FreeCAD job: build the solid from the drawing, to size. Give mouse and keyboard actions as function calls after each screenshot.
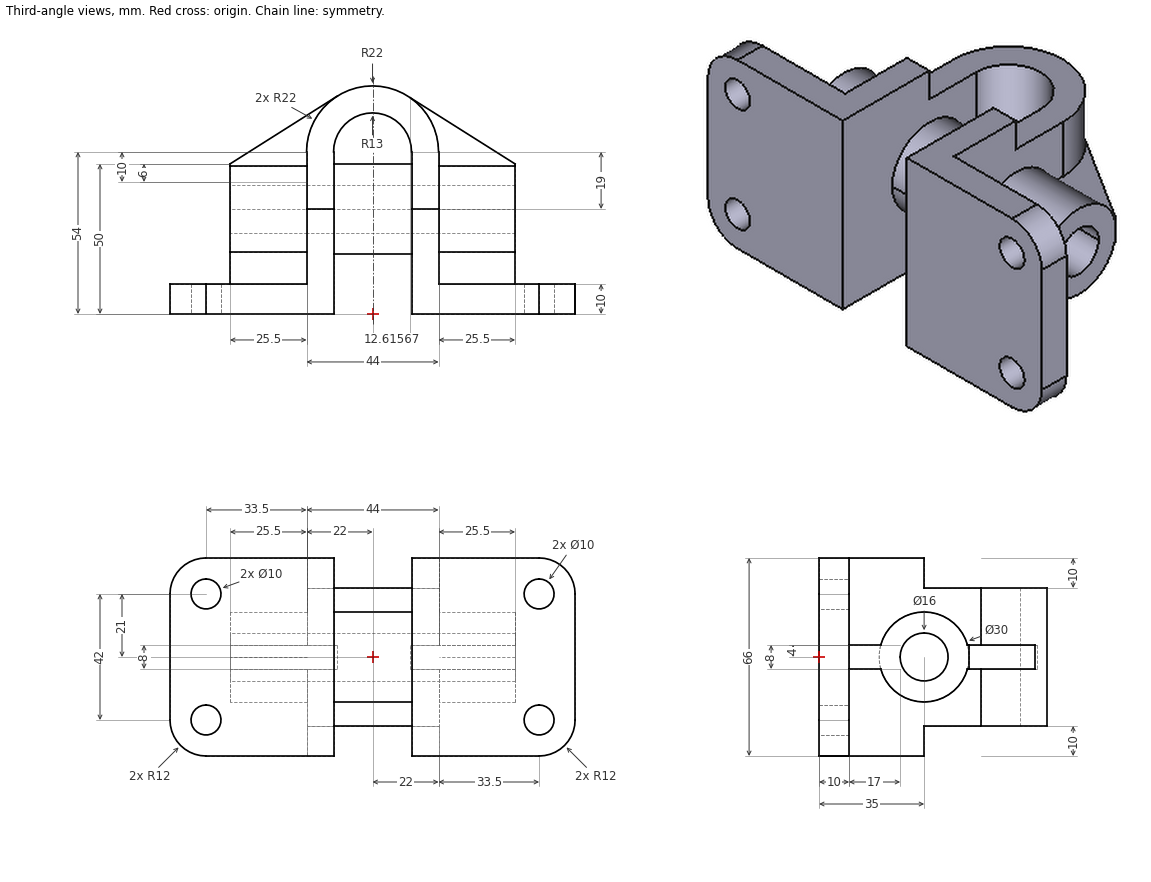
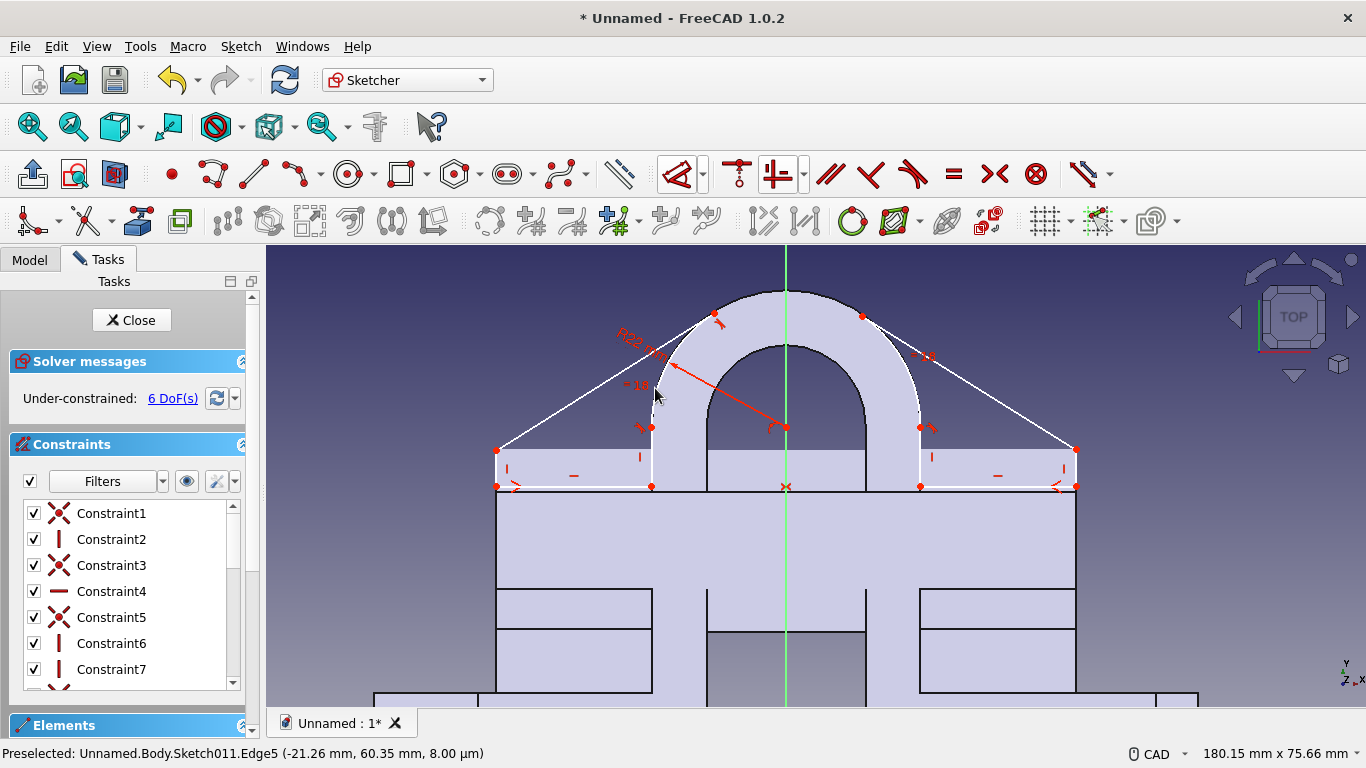
scroll(496, 462, up, 2)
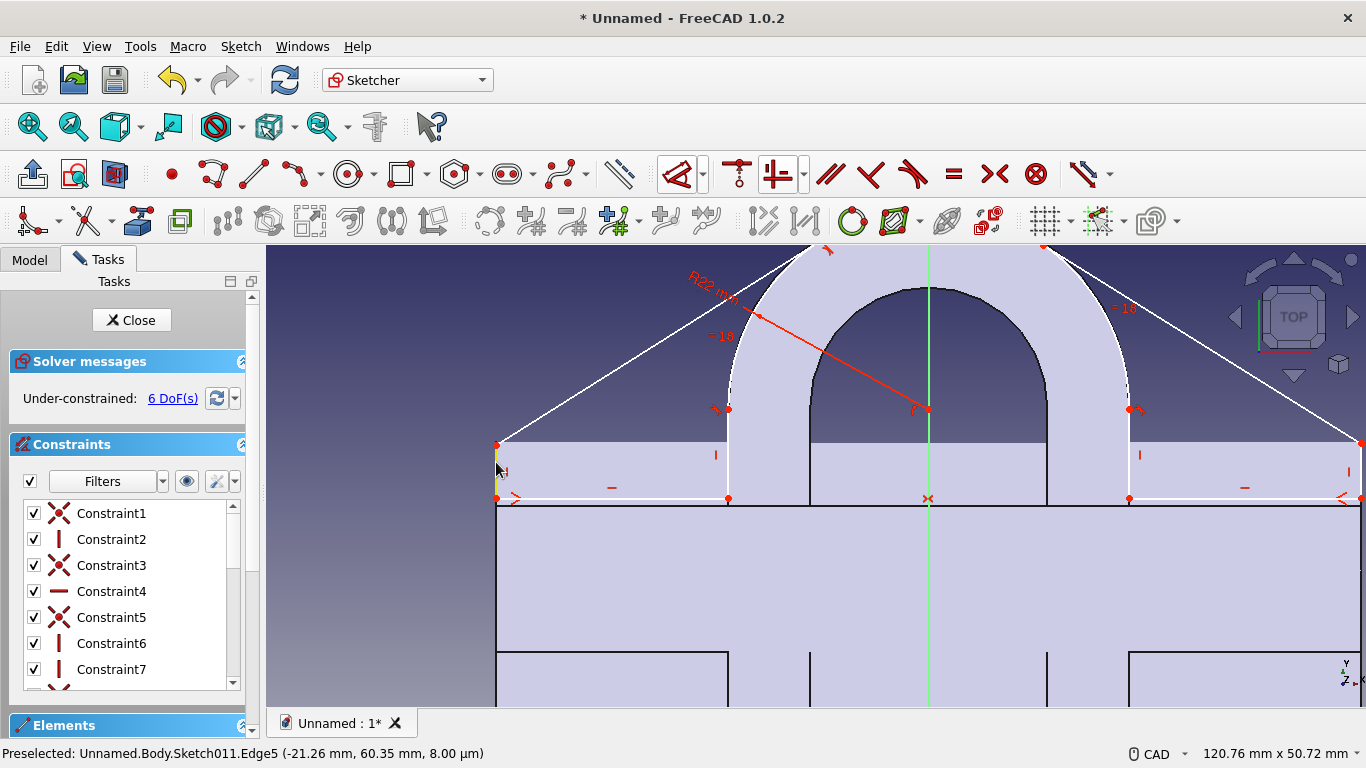
click(496, 461)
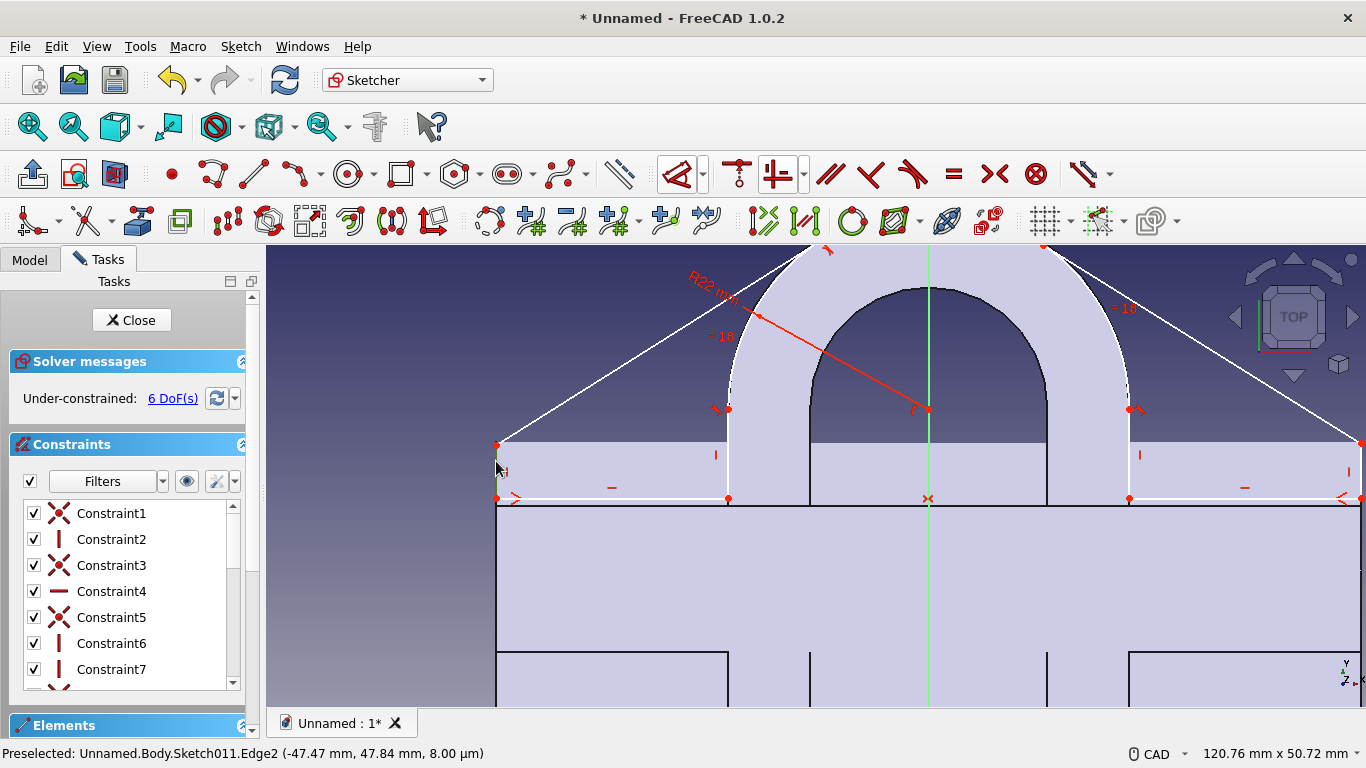
click(702, 174)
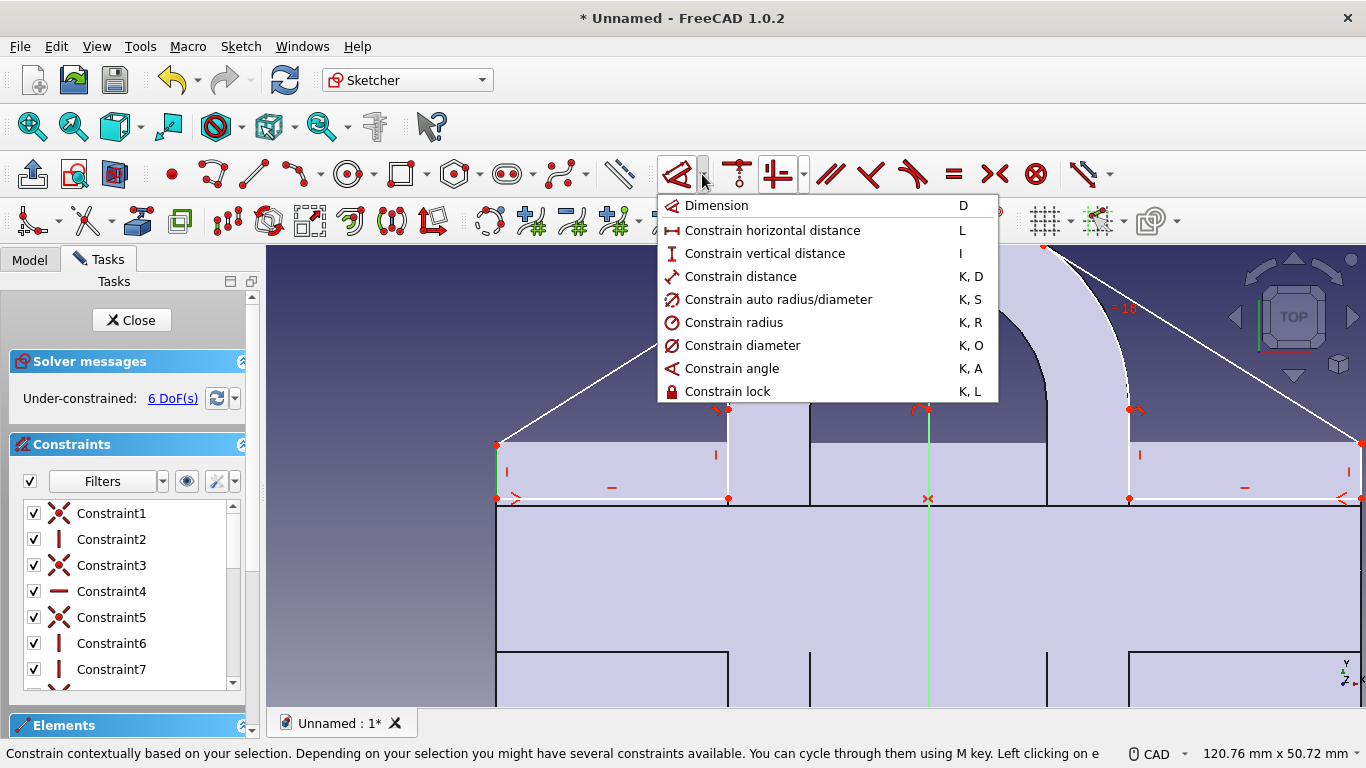
click(828, 254)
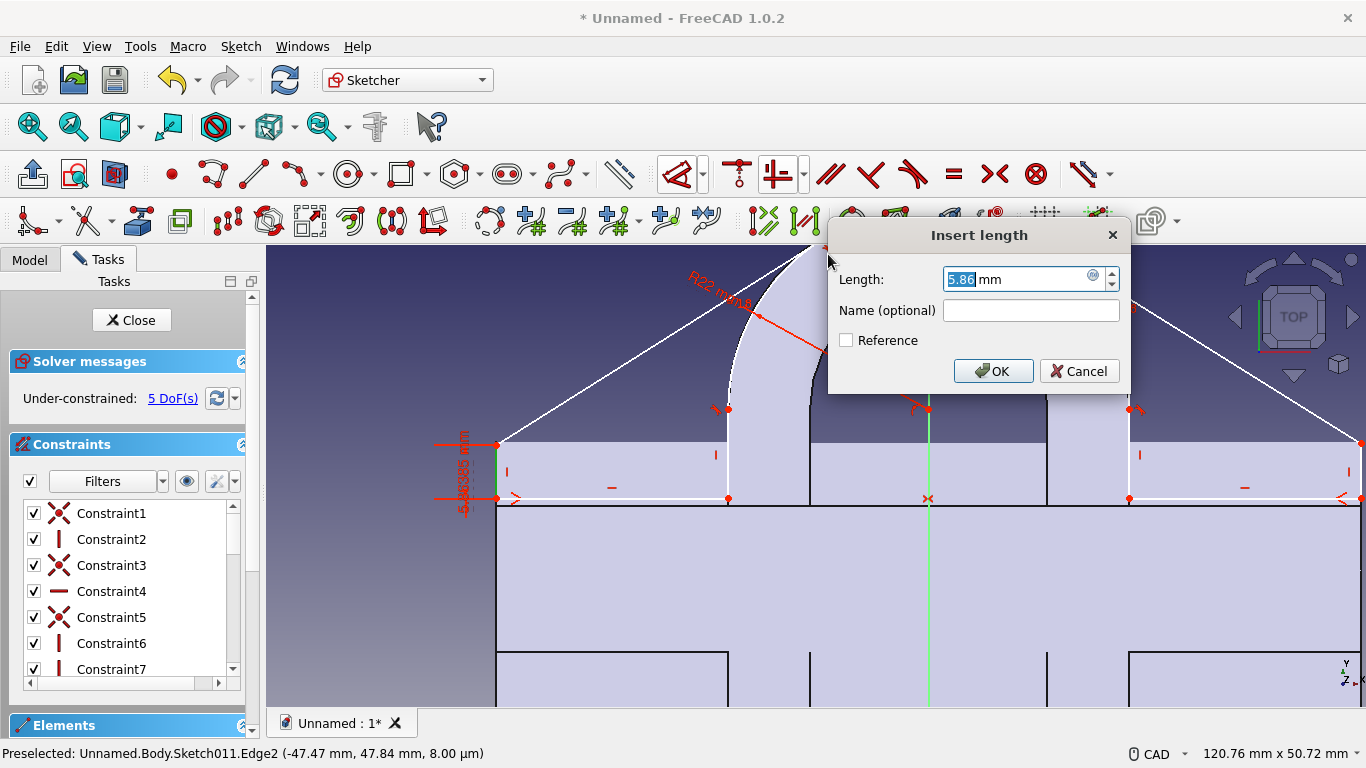
text(6)
key(Return)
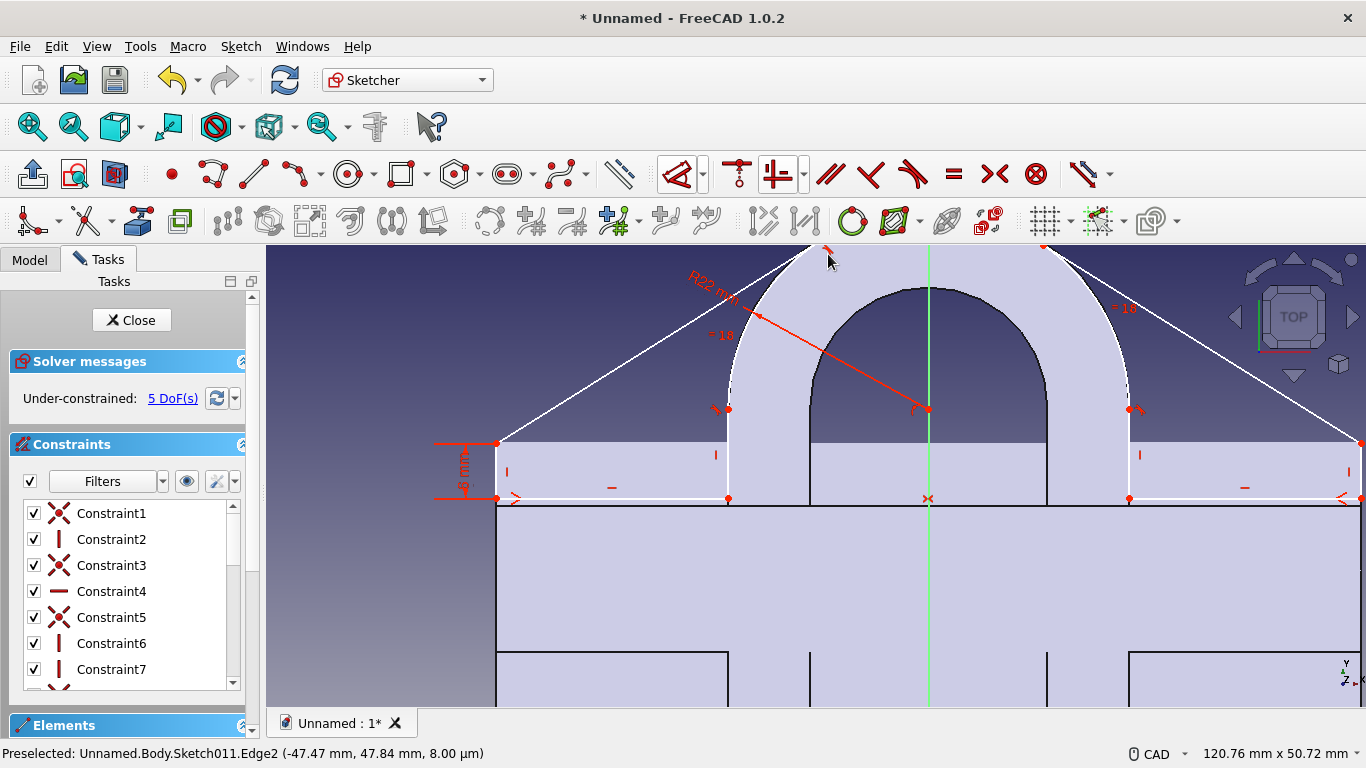
scroll(600, 402, down, 4)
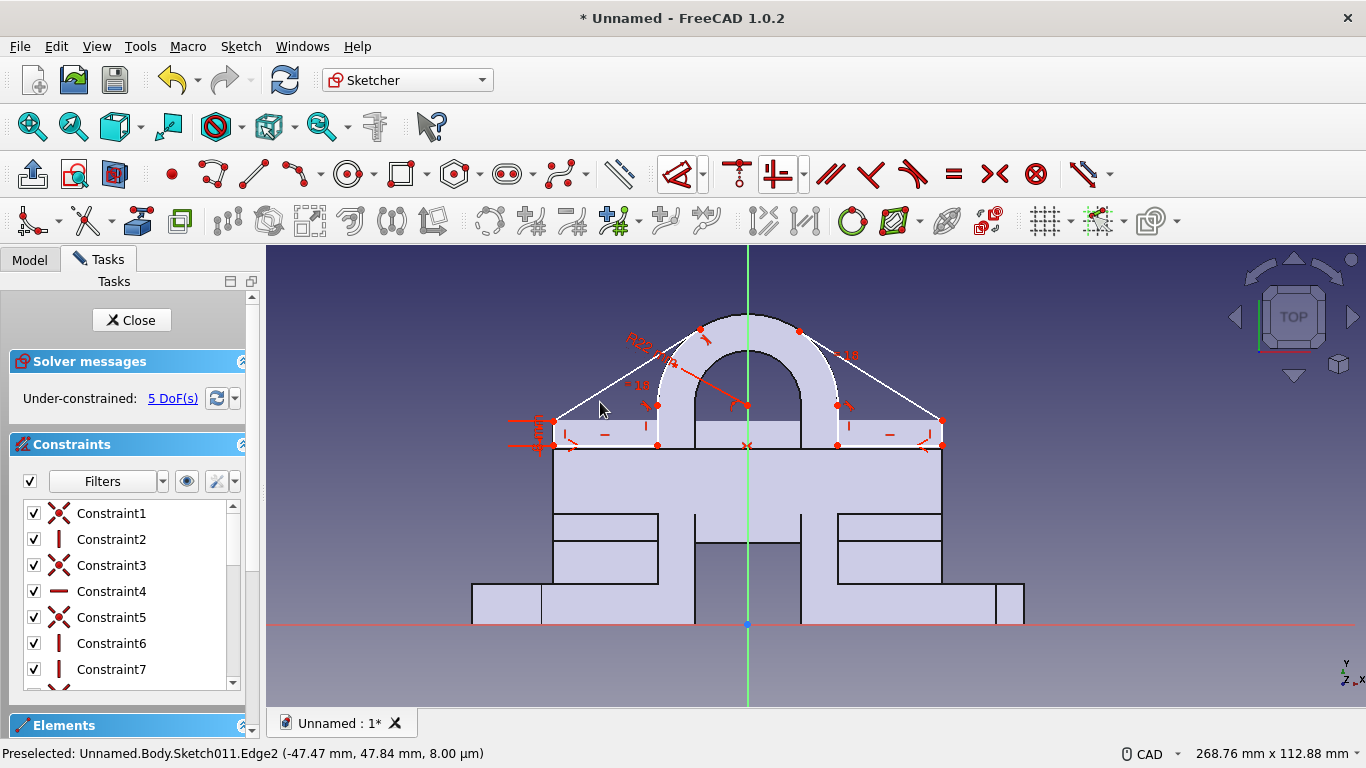
scroll(942, 438, up, 4)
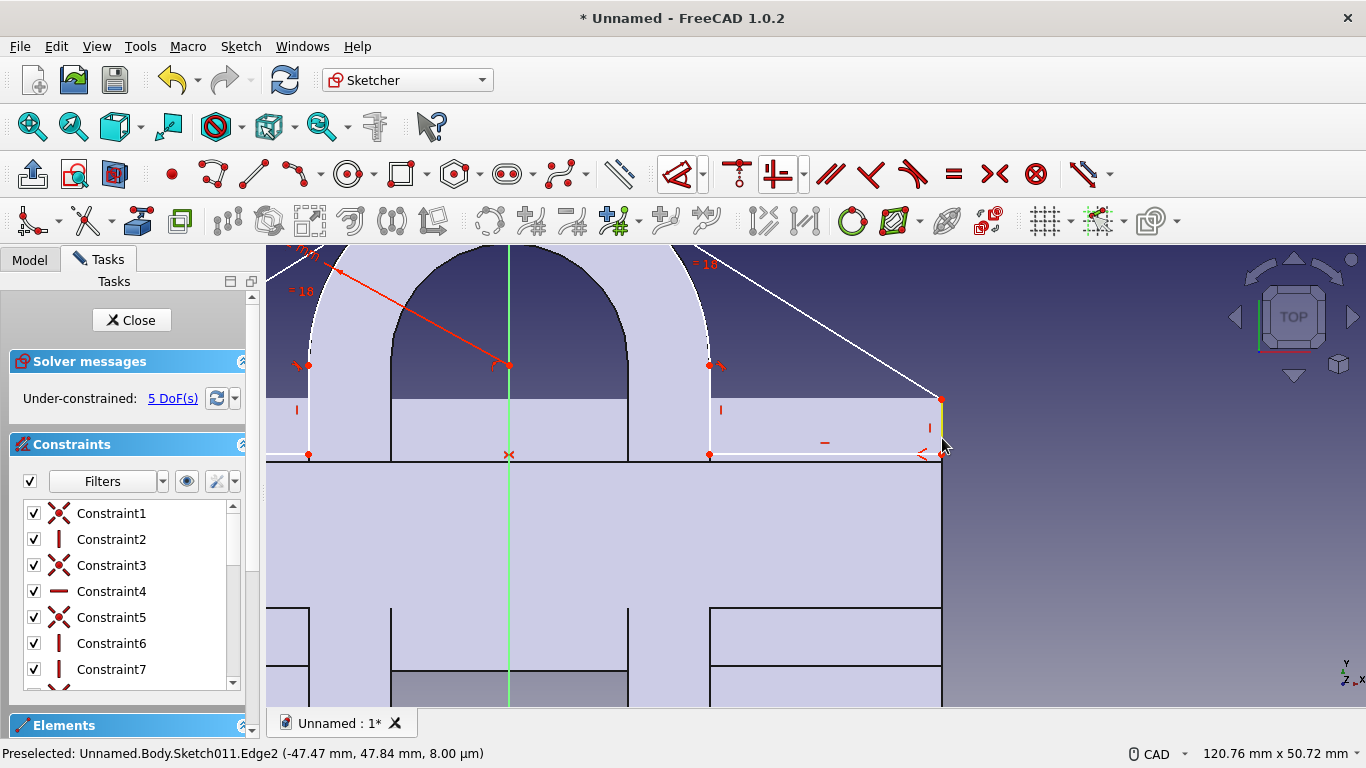
click(942, 438)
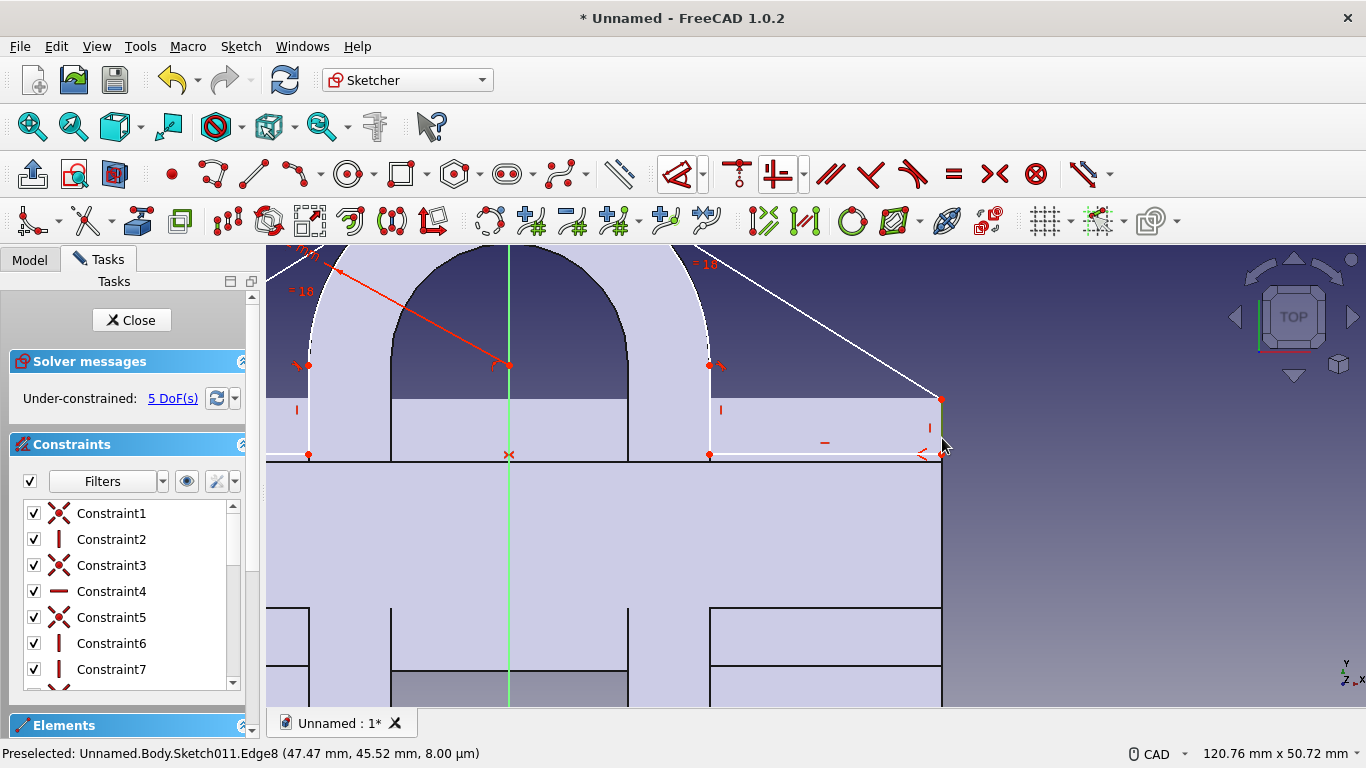
click(702, 174)